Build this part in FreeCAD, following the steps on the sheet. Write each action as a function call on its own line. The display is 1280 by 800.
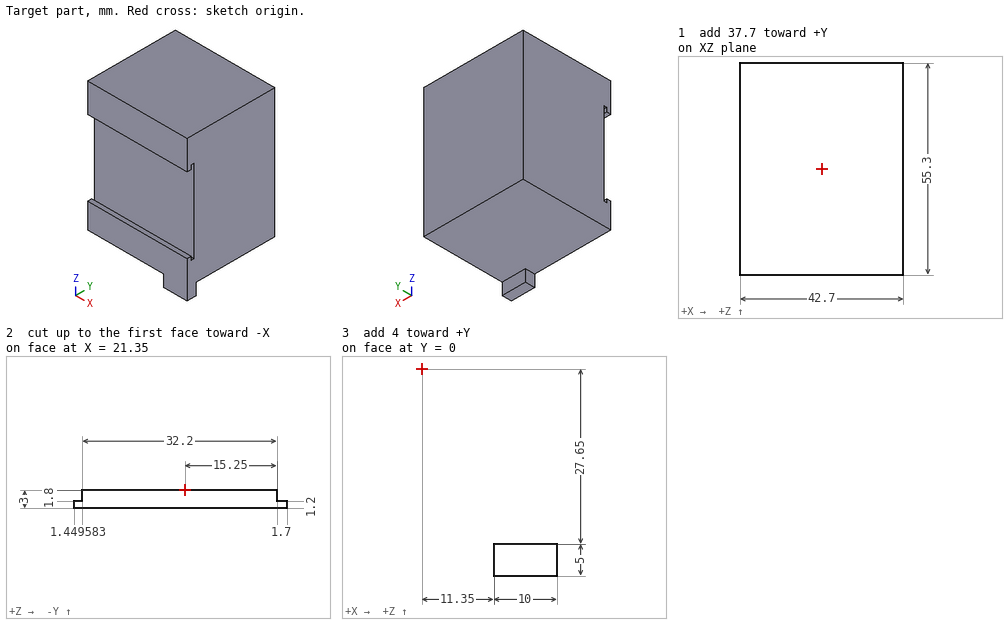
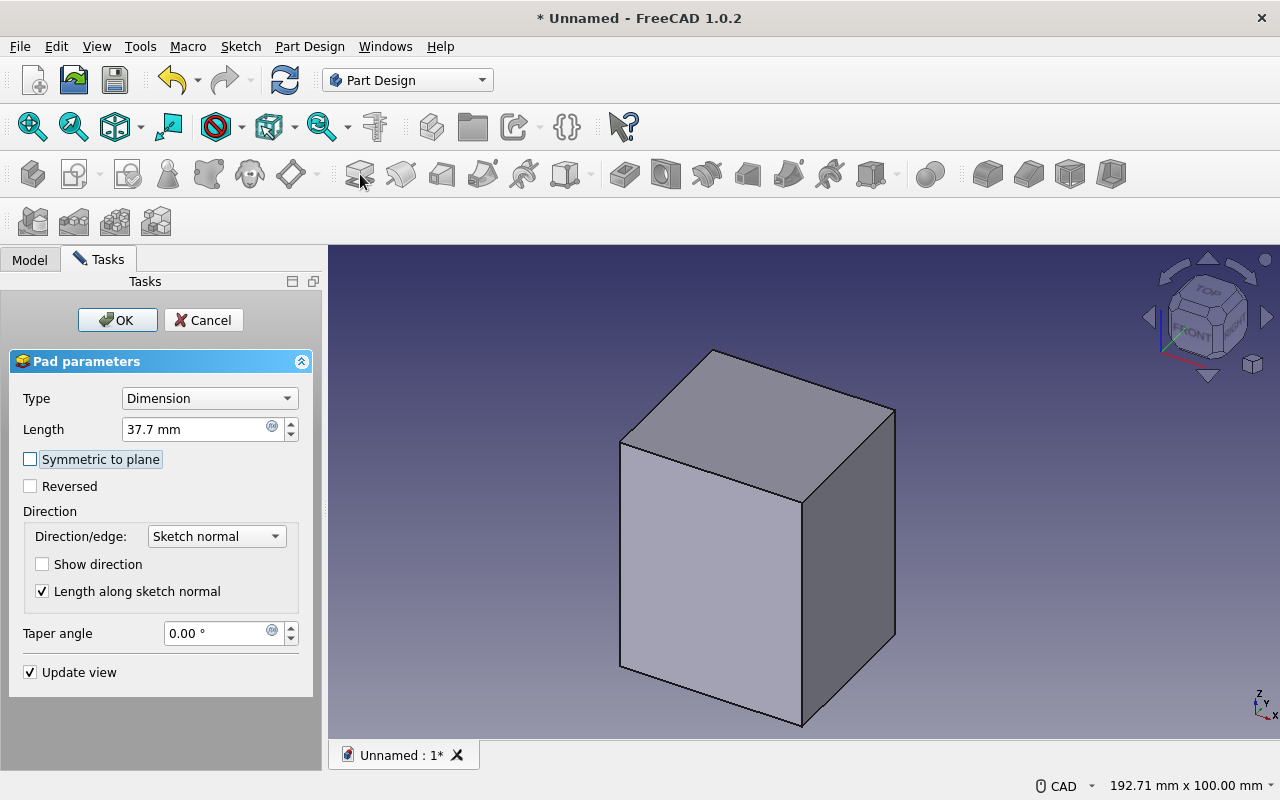
click(31, 486)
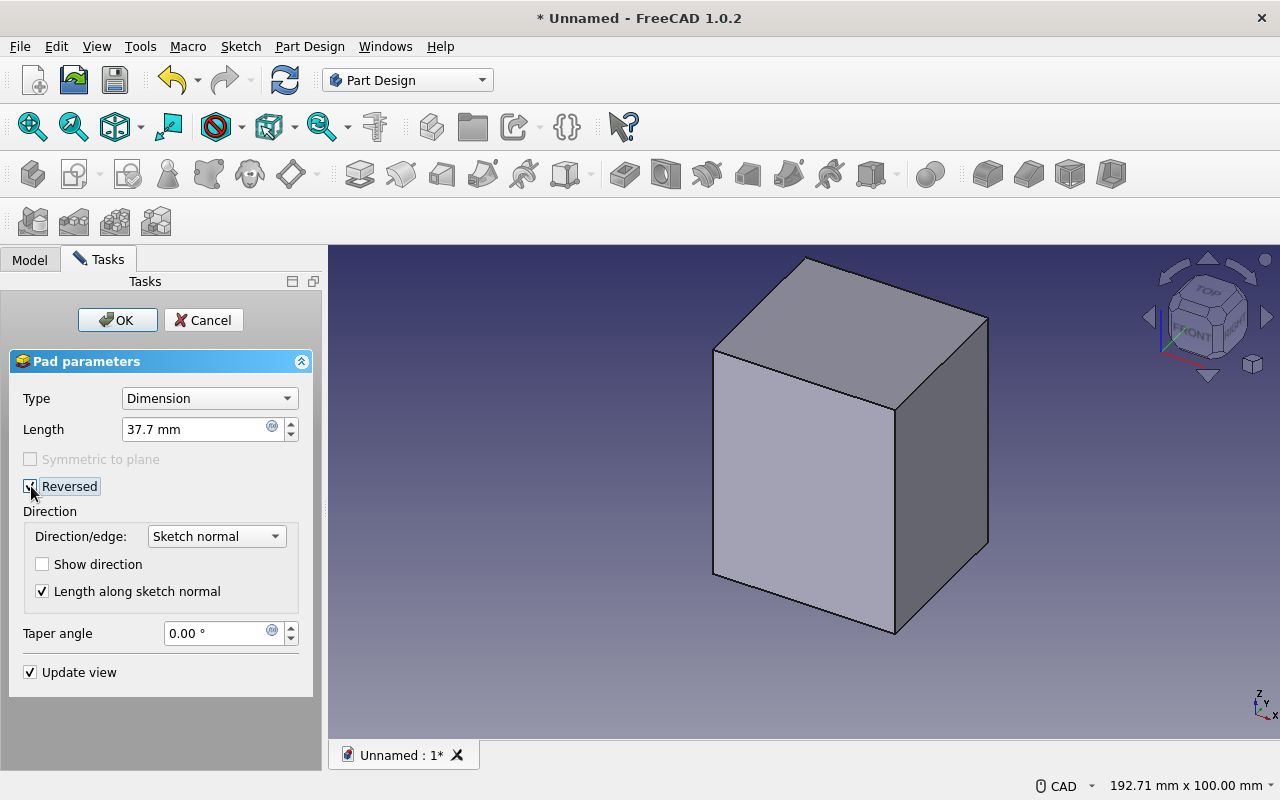
click(118, 320)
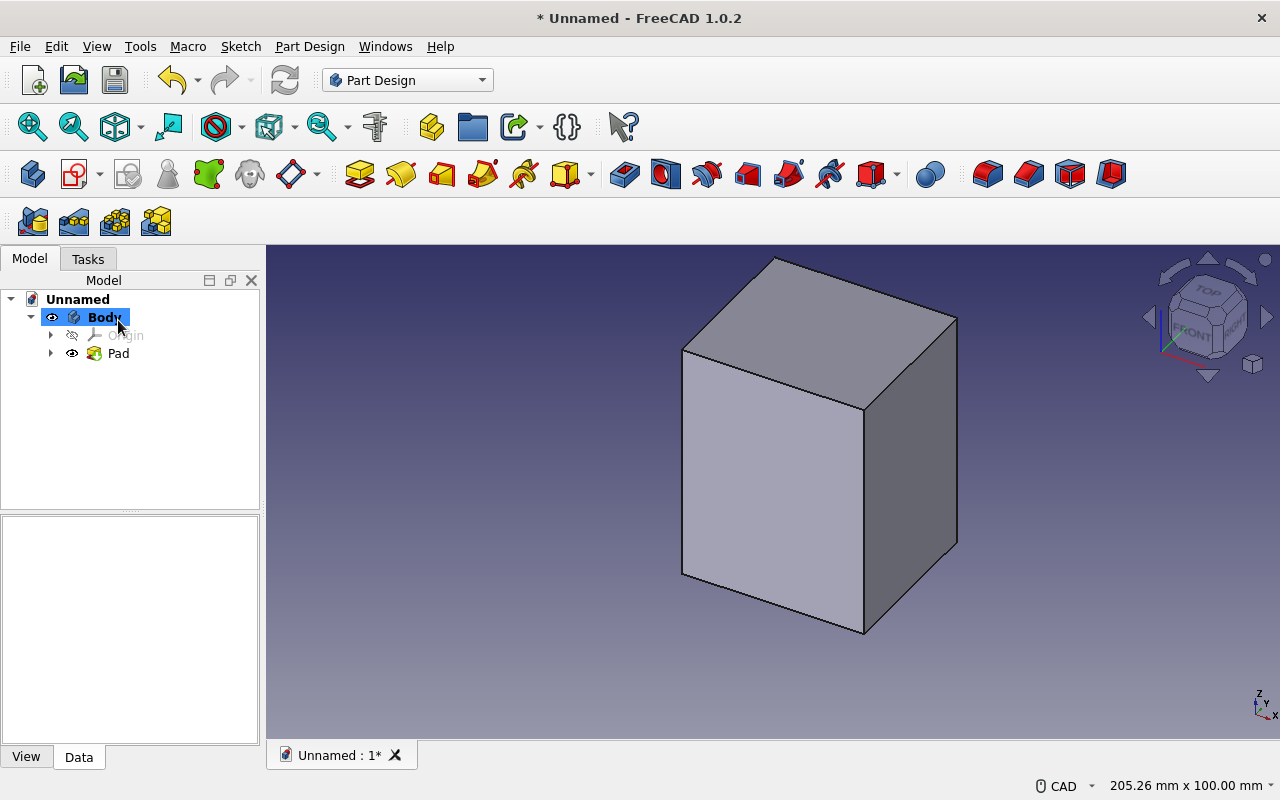
click(911, 475)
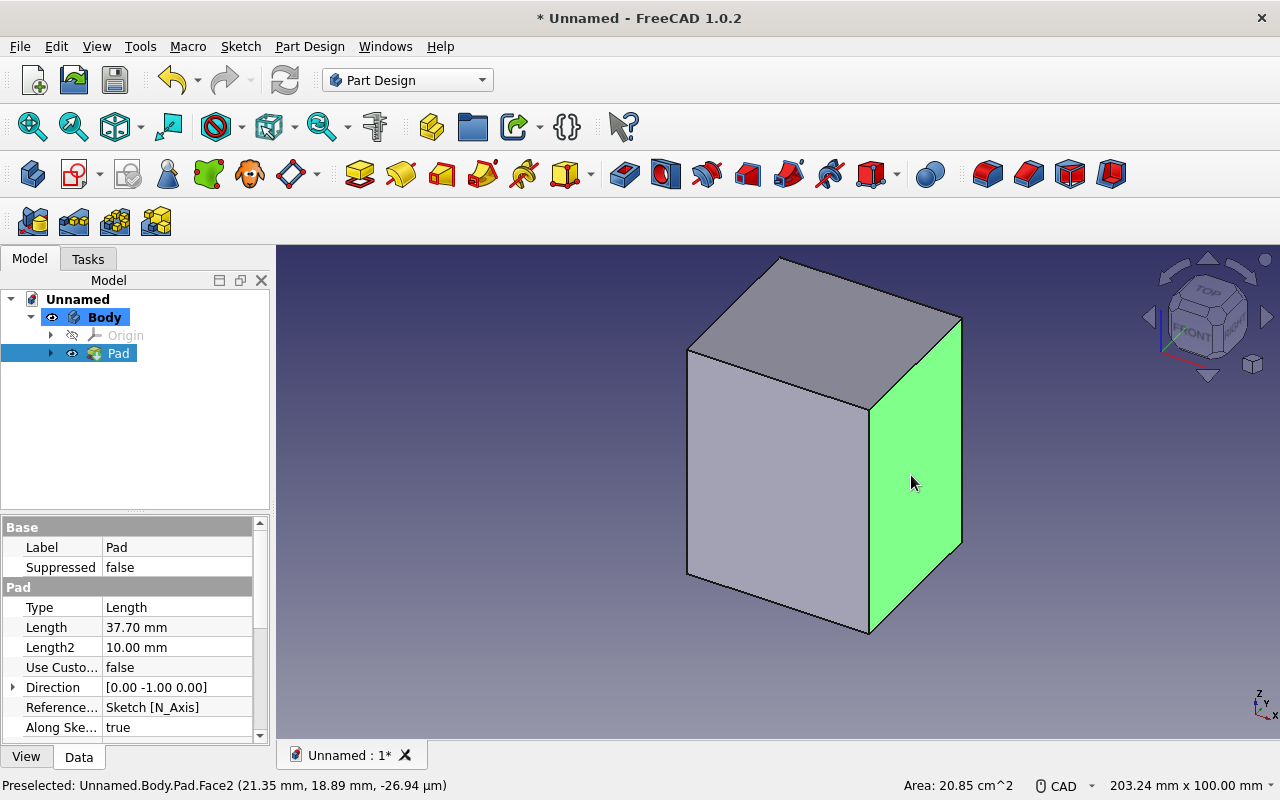
click(74, 174)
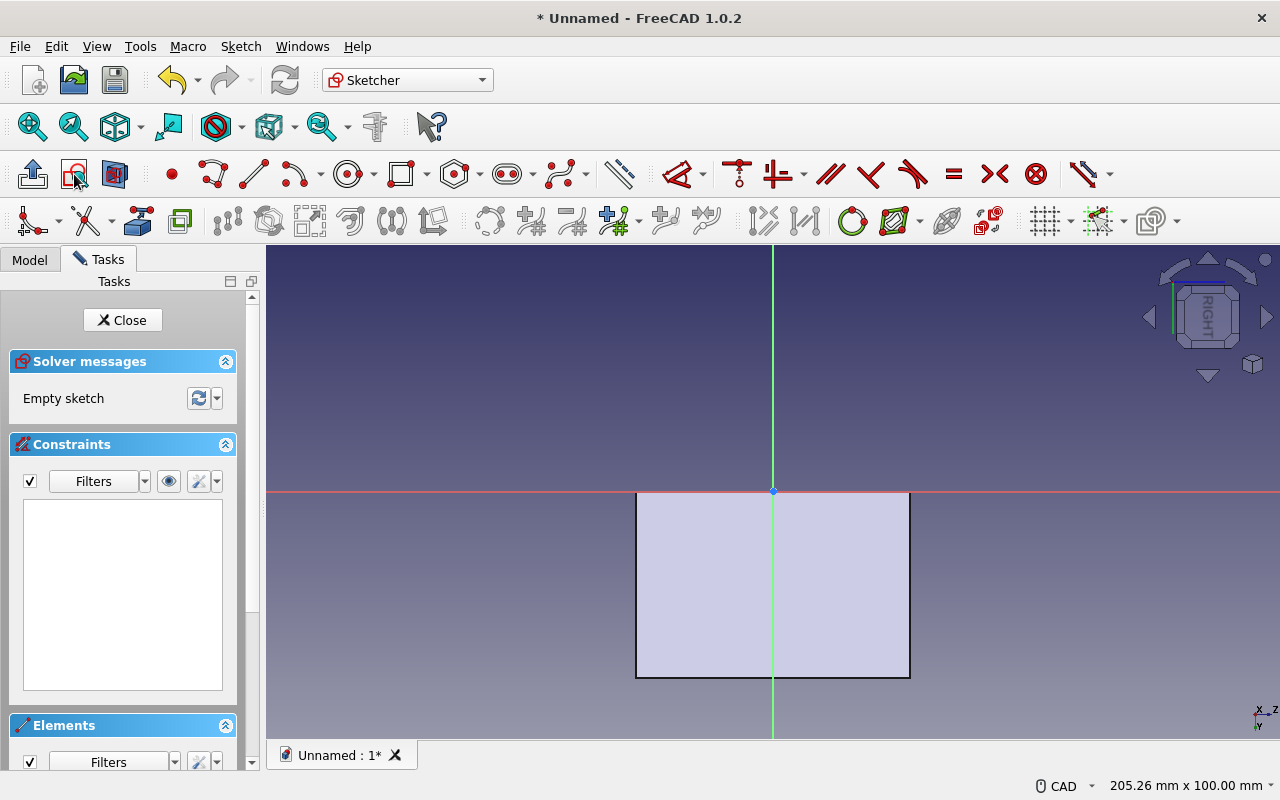
scroll(797, 503, up, 6)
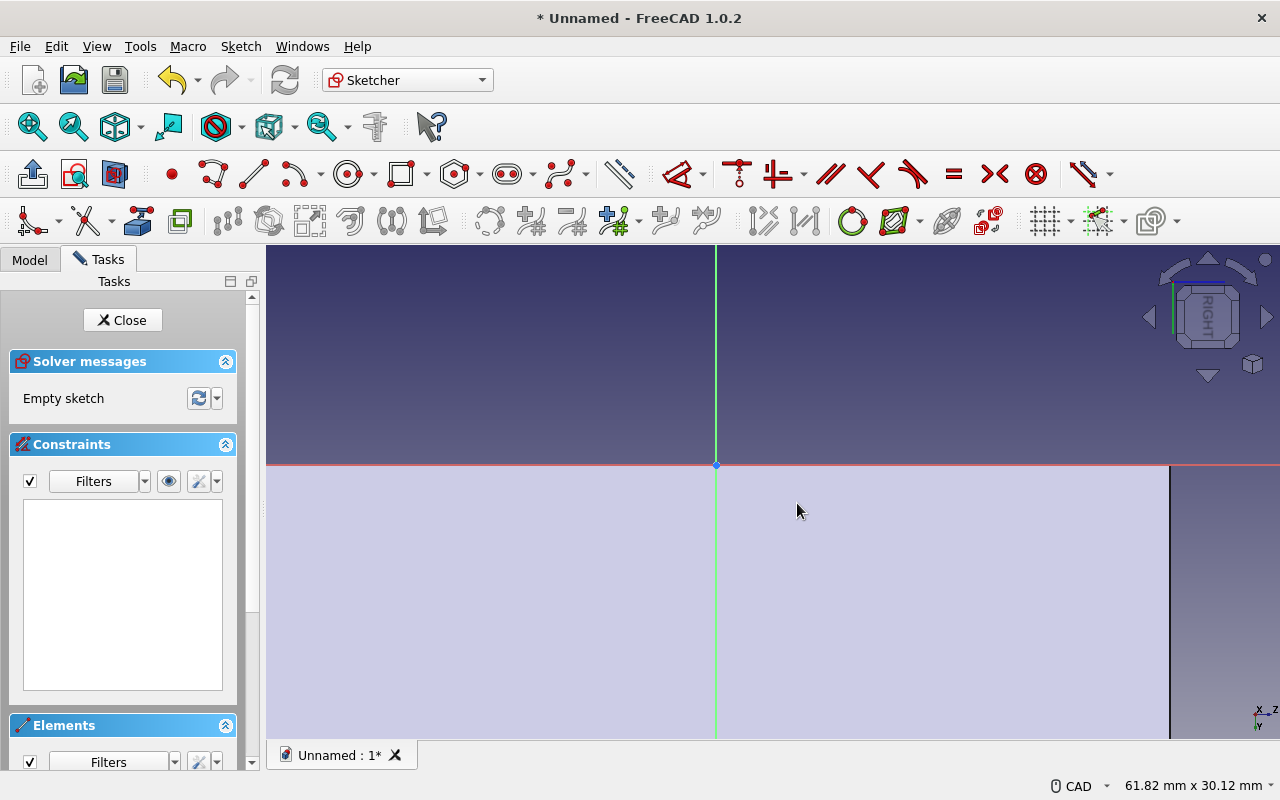
key(g)
key(m)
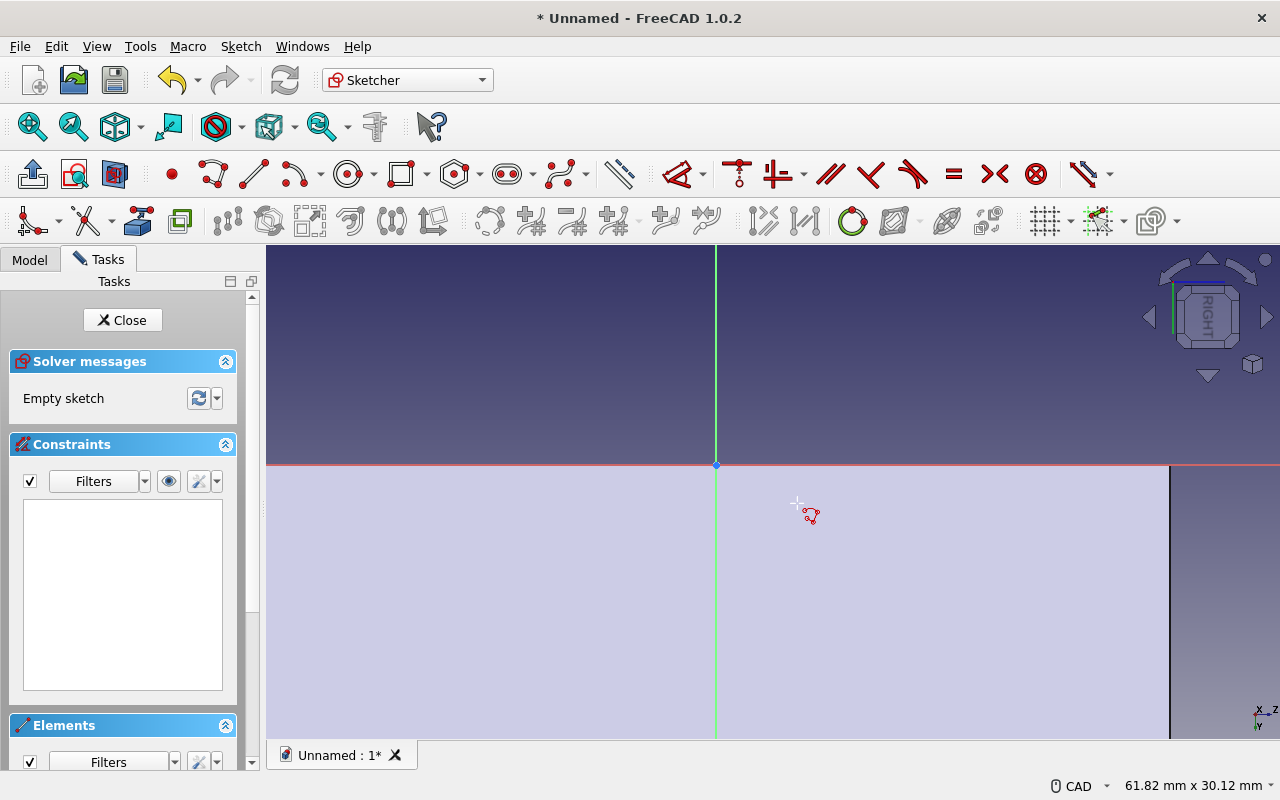
click(966, 465)
click(438, 474)
click(438, 495)
click(414, 495)
click(414, 514)
click(994, 514)
click(994, 495)
click(966, 495)
click(966, 465)
key(Escape)
key(Escape)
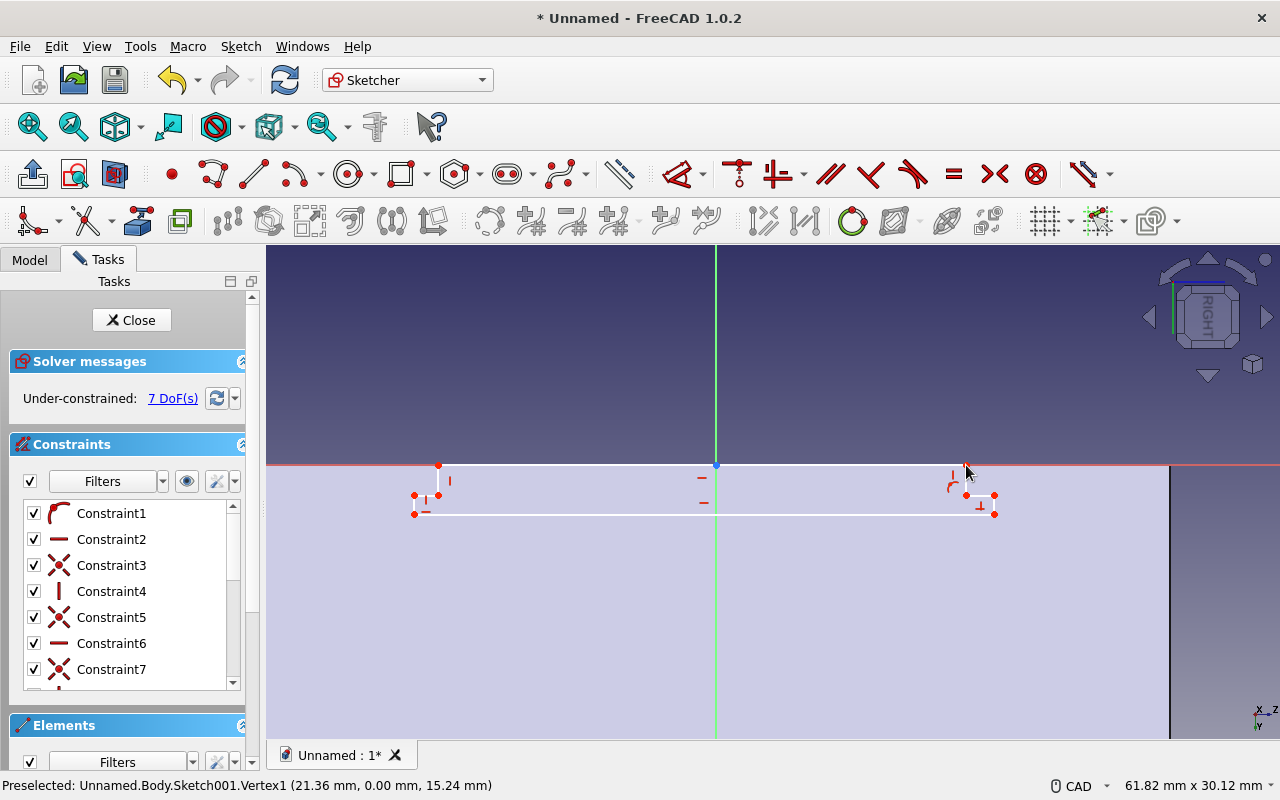
click(676, 174)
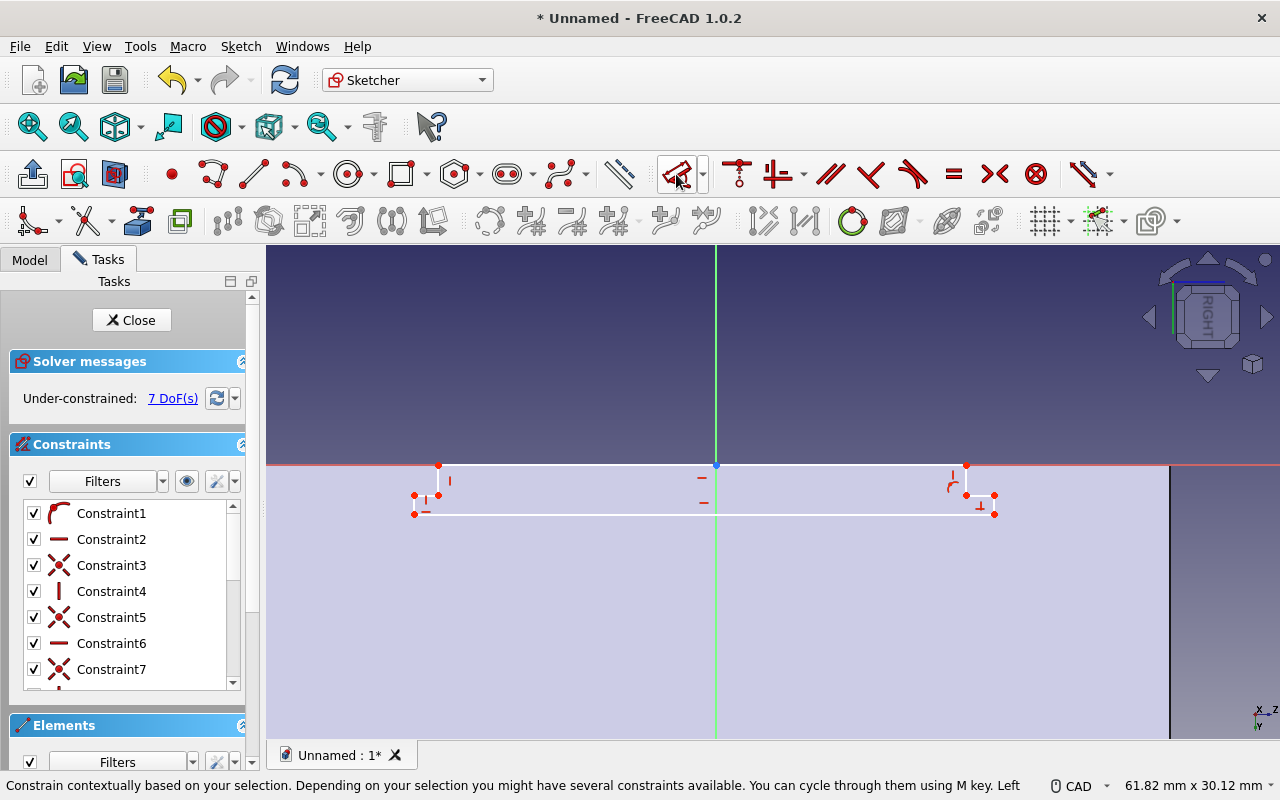
click(414, 515)
click(380, 490)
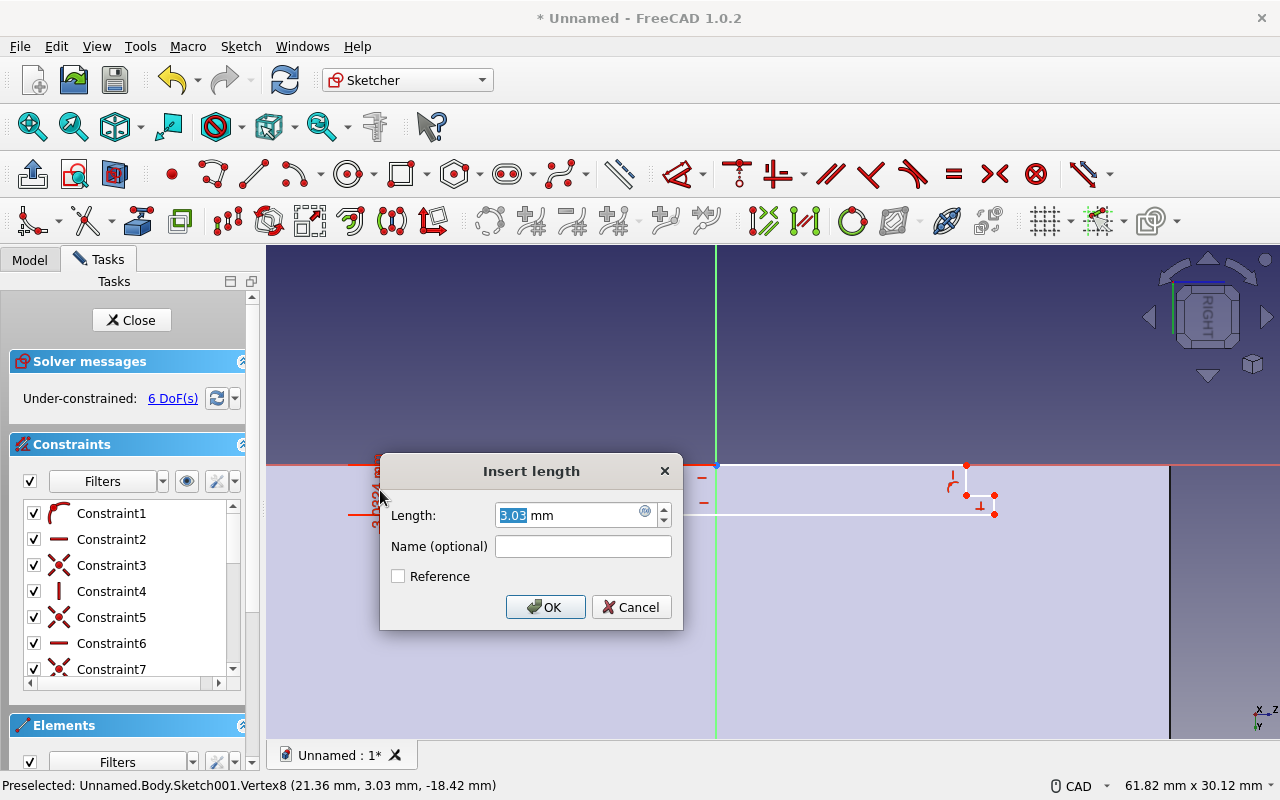
text(3)
key(Return)